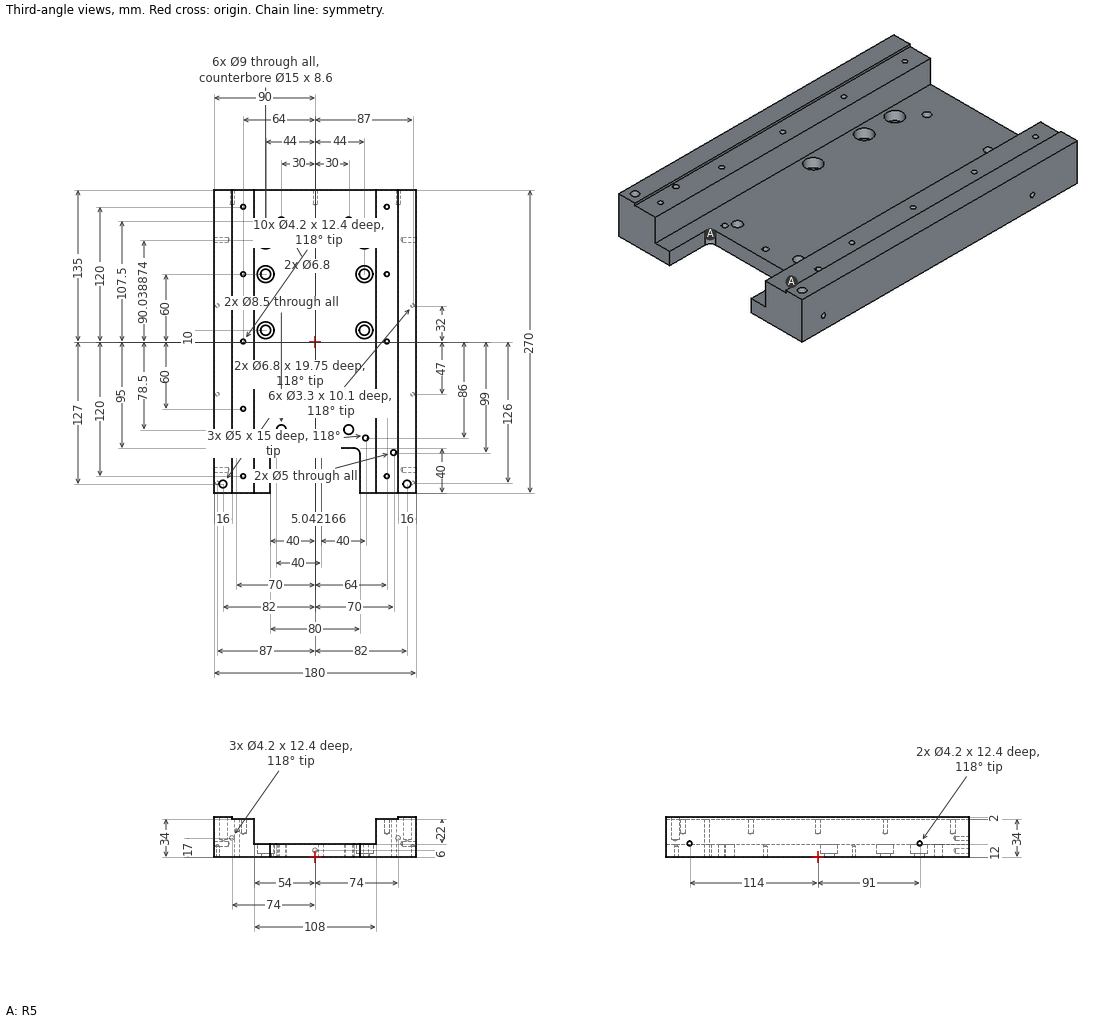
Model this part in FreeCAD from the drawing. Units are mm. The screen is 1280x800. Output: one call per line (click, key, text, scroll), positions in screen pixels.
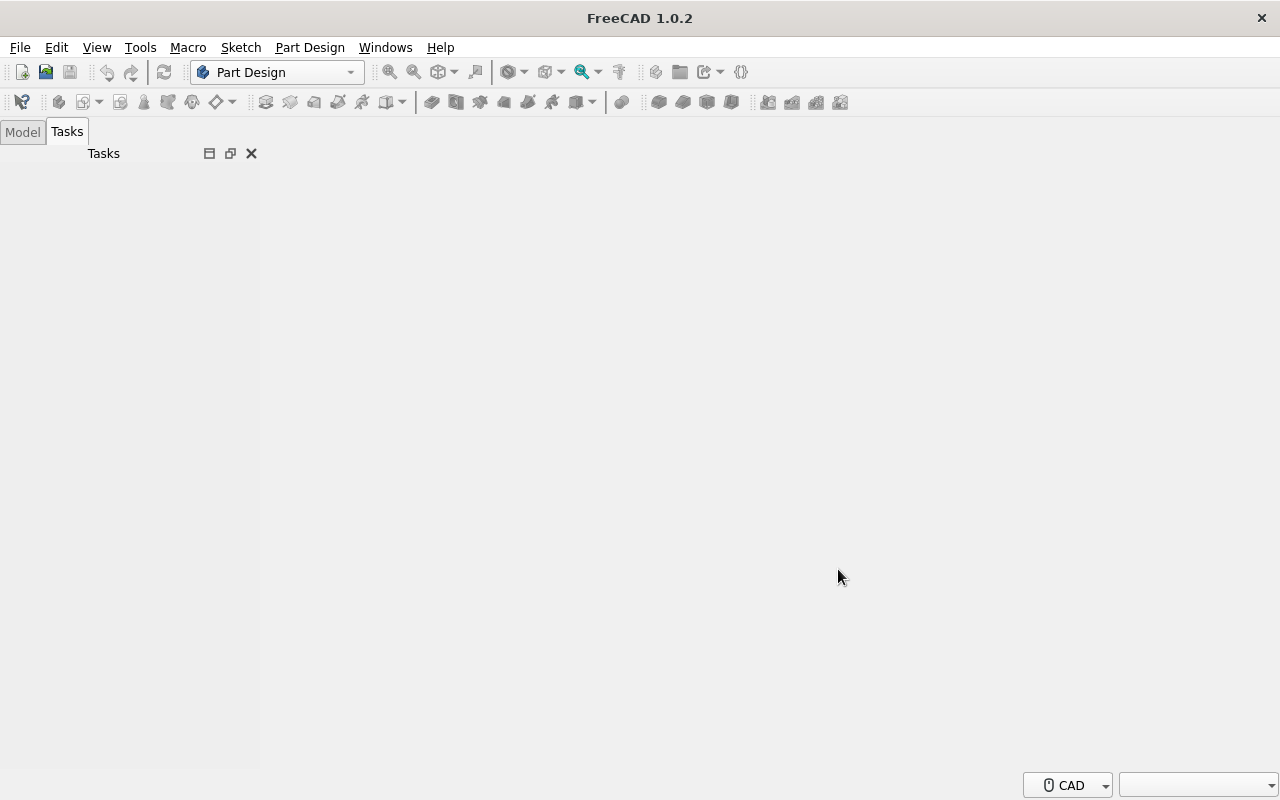
click(22, 72)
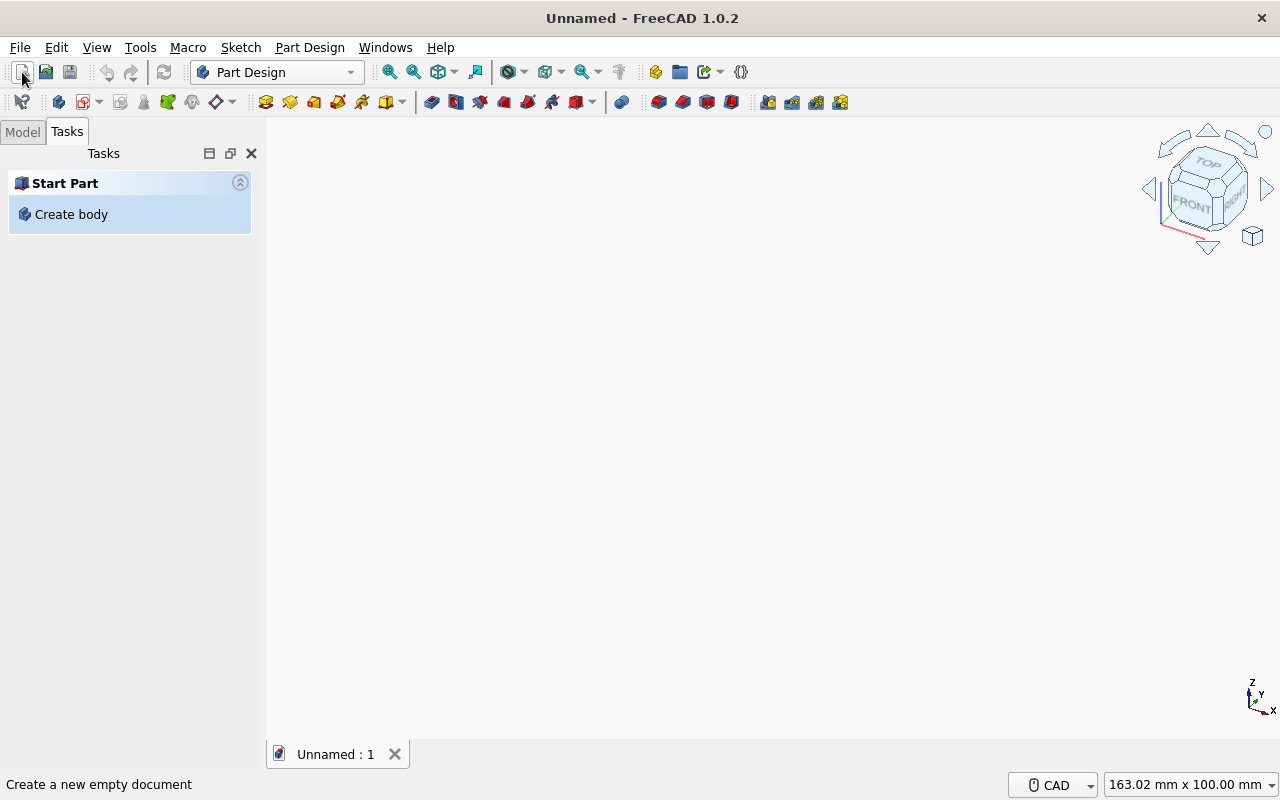
click(84, 102)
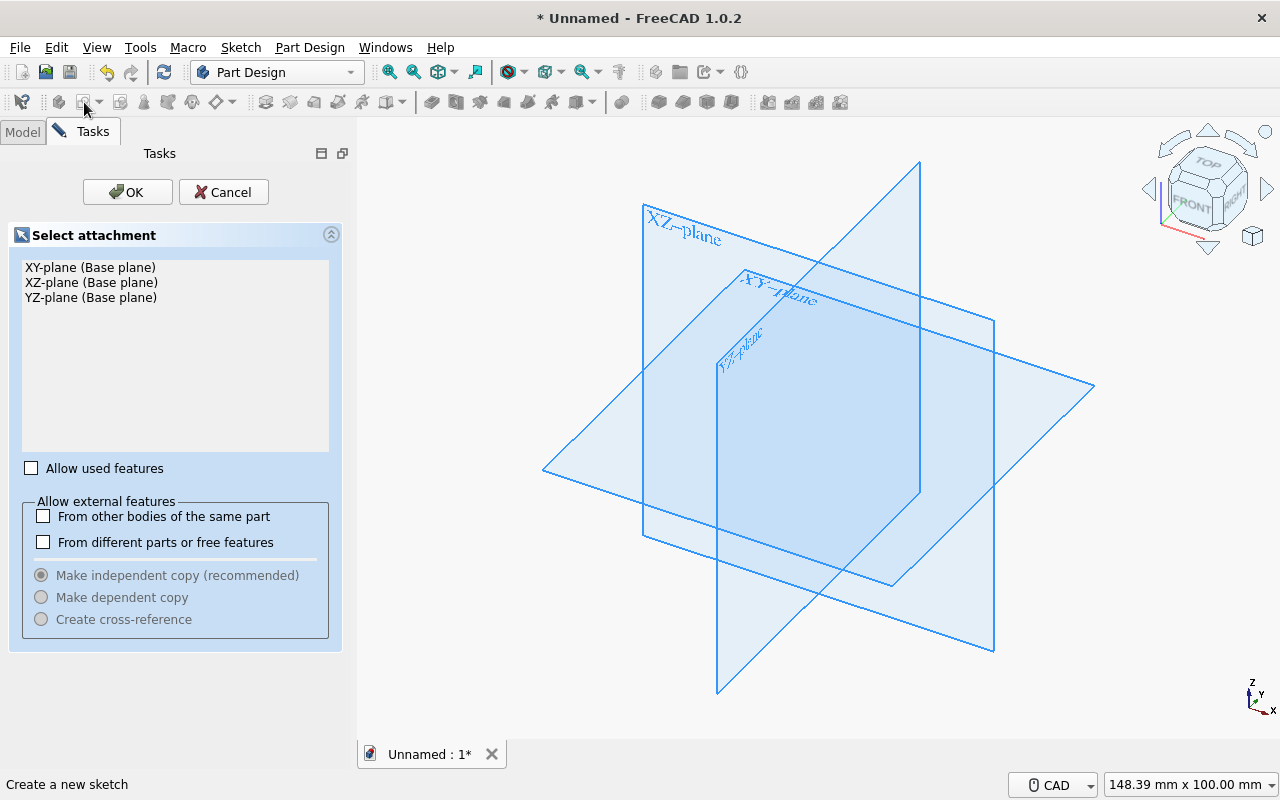
click(82, 268)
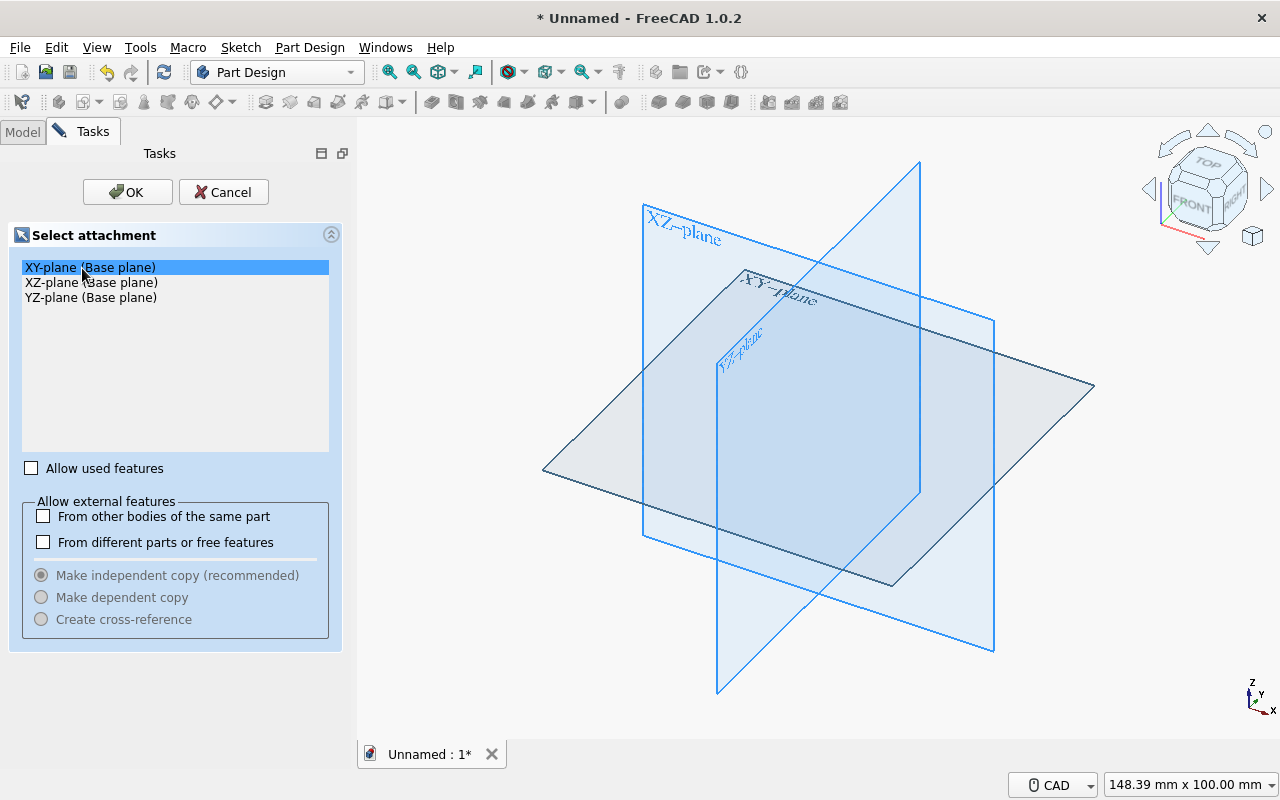
click(128, 192)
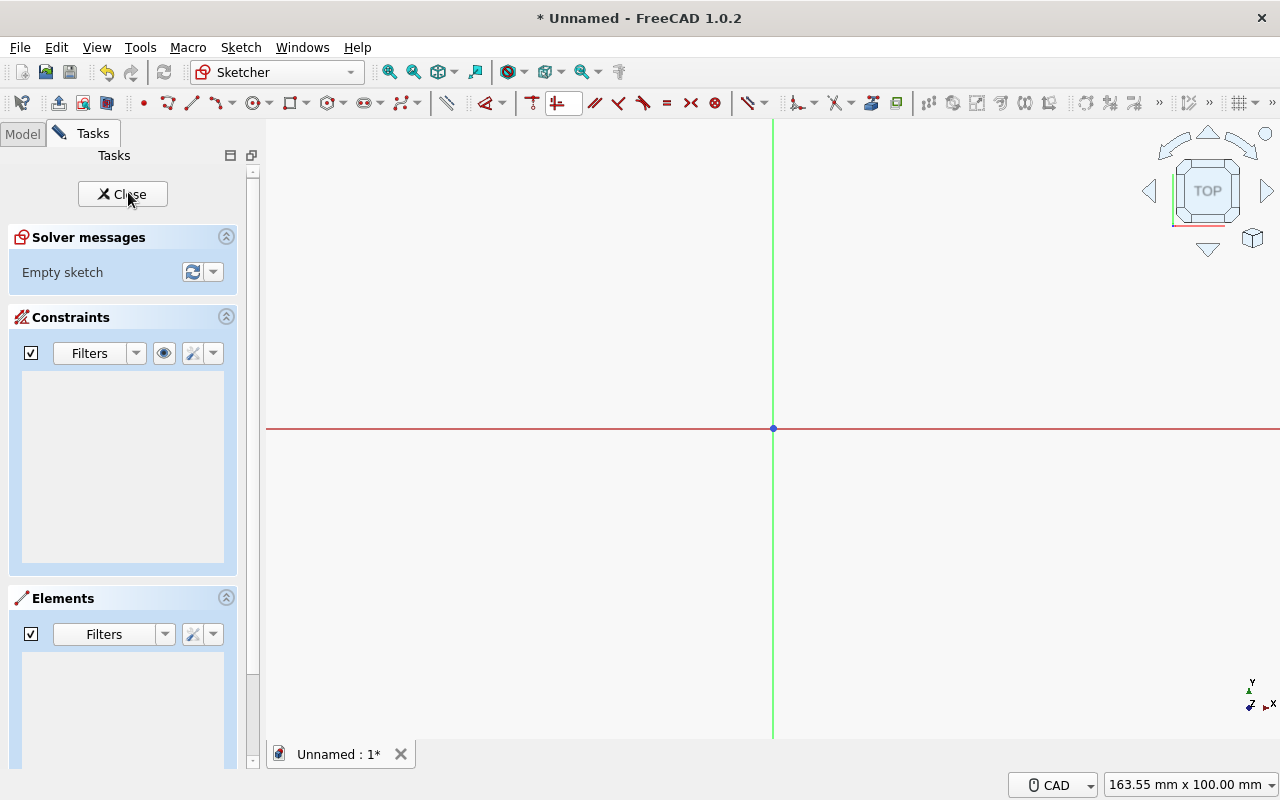
scroll(682, 429, down, 7)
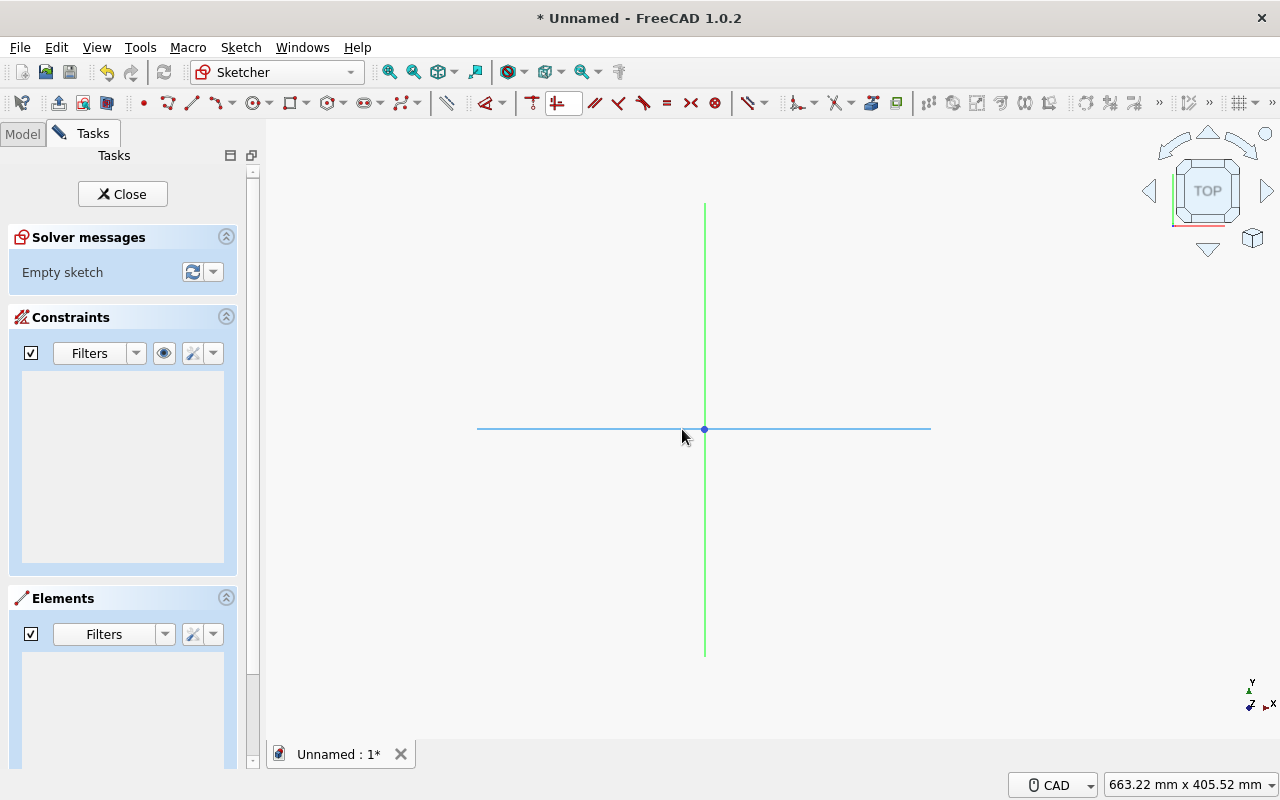
click(308, 104)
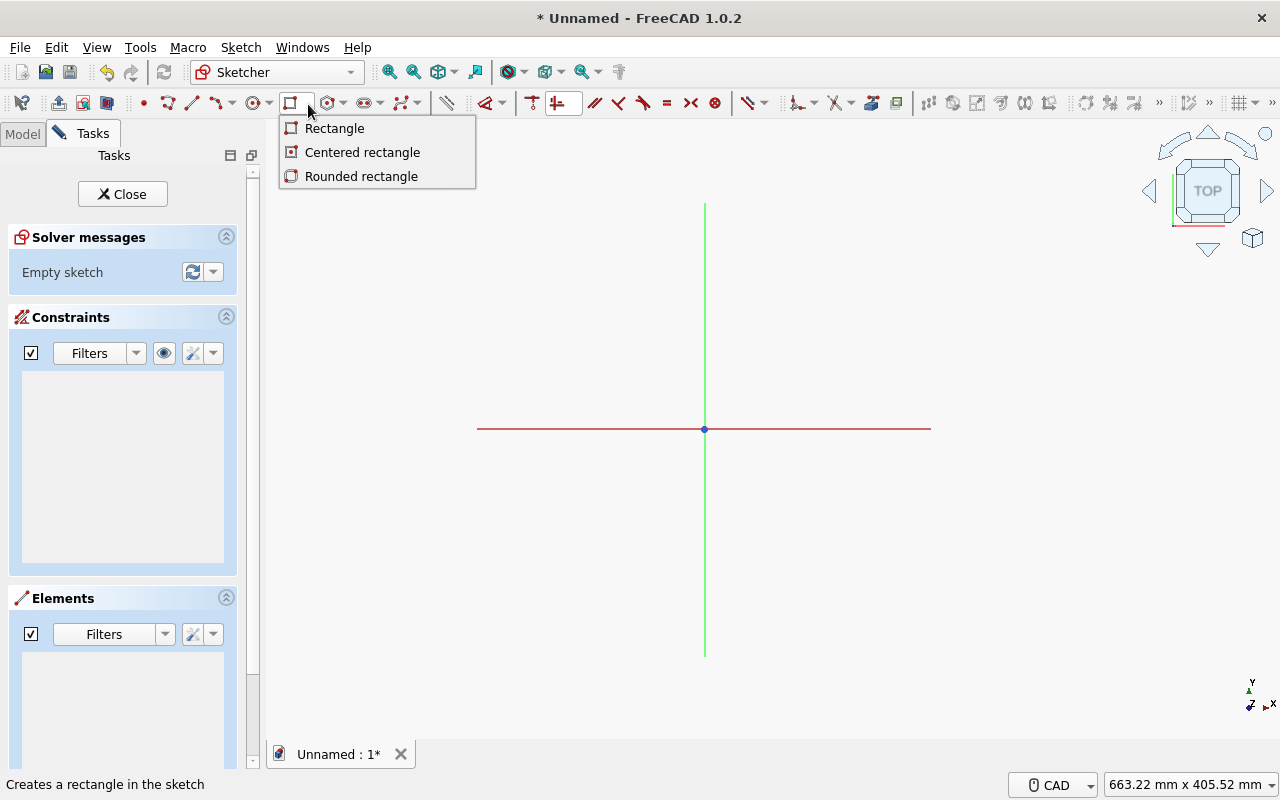
click(378, 152)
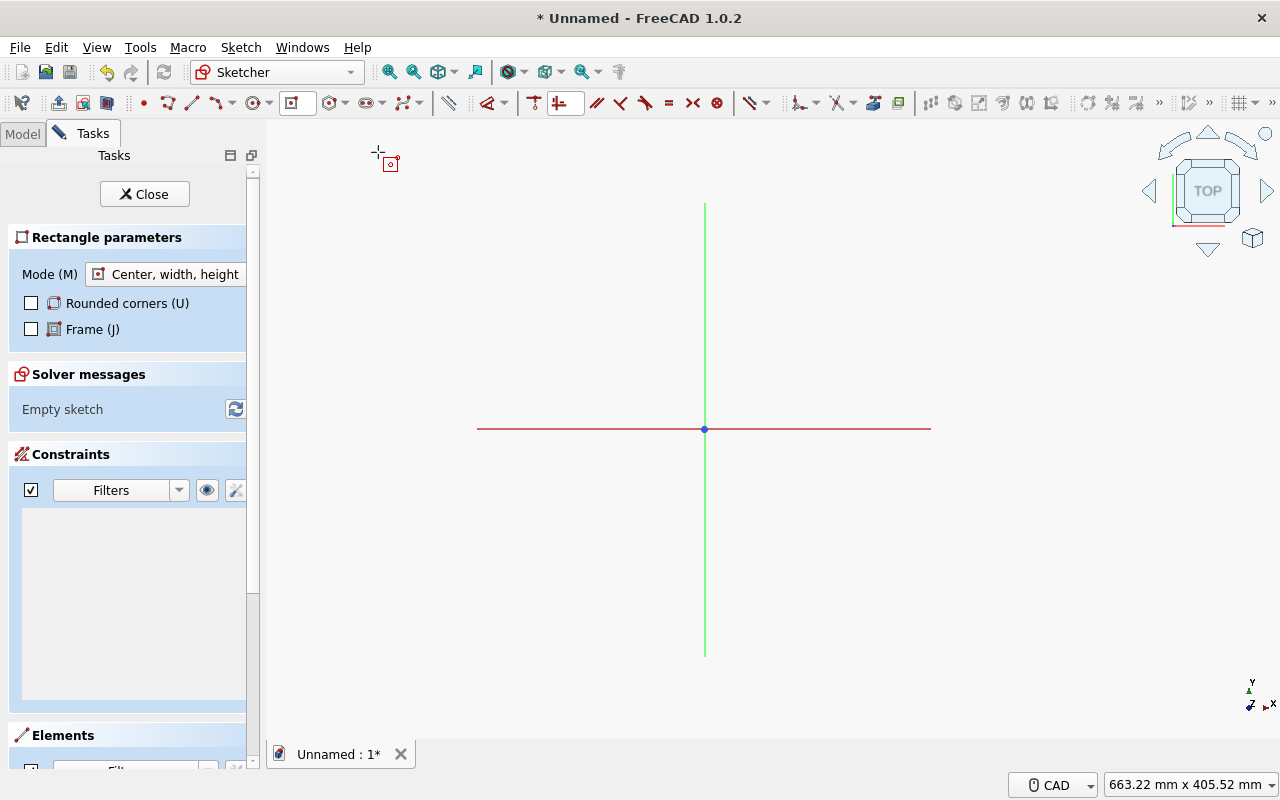
click(705, 429)
move(842, 223)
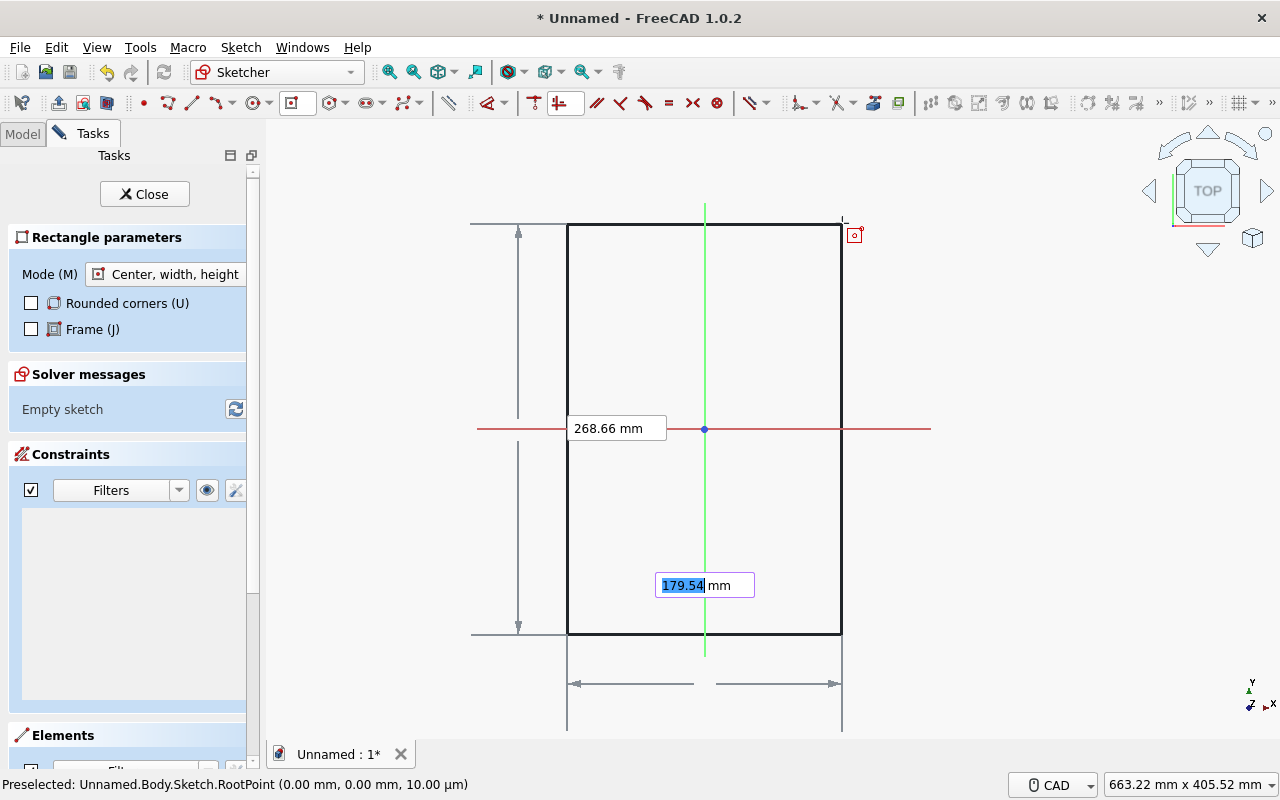
text(180)
key(Tab)
text(270)
key(Return)
key(Escape)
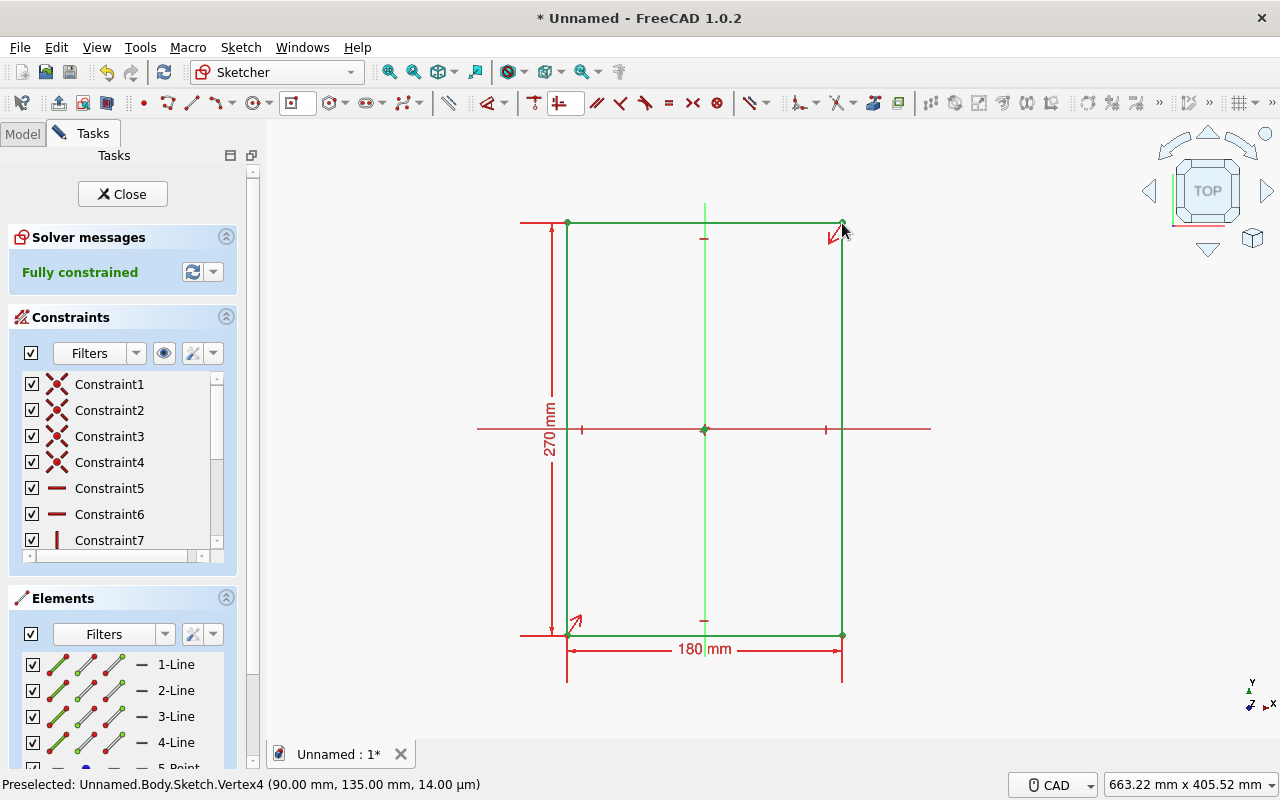
click(123, 194)